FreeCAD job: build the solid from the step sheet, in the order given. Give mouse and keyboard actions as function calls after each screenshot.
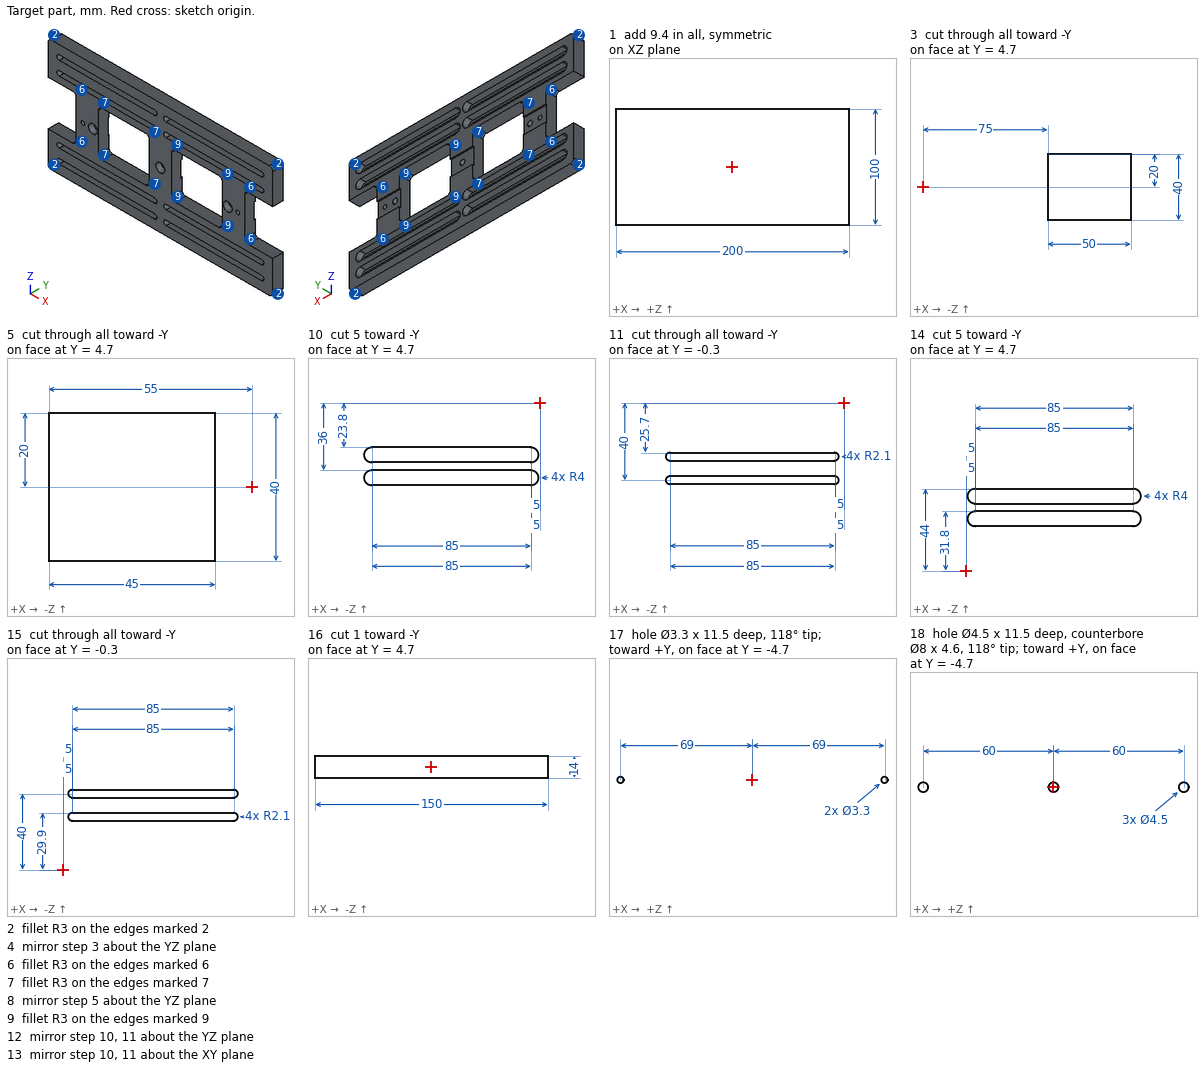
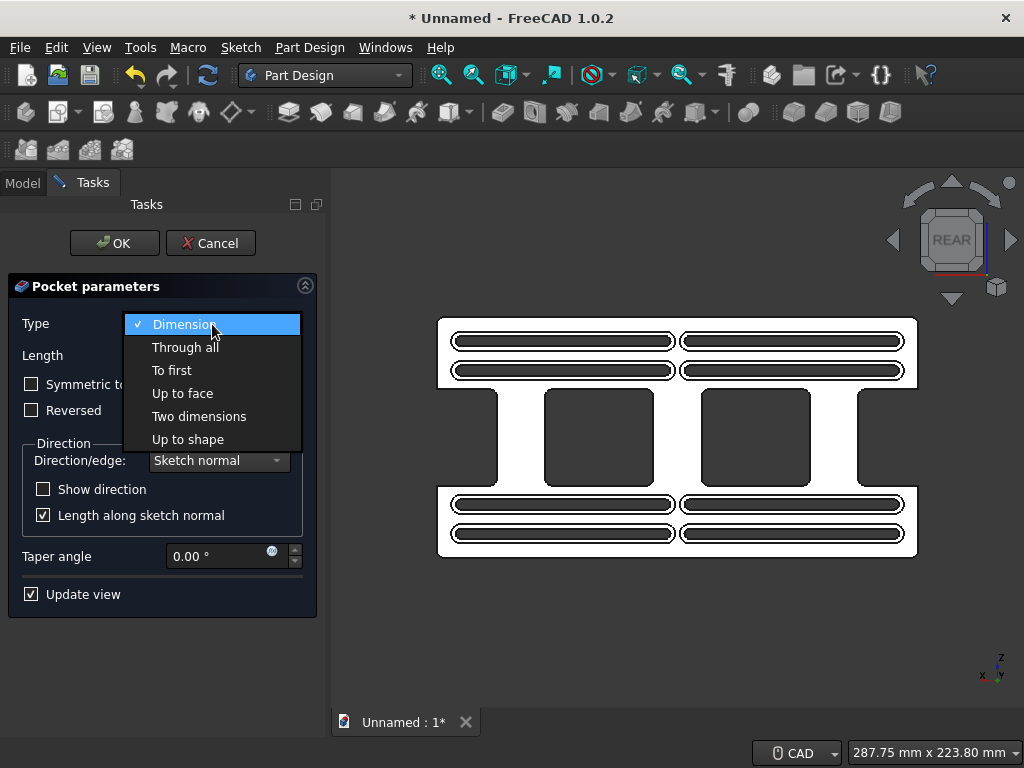
click(212, 348)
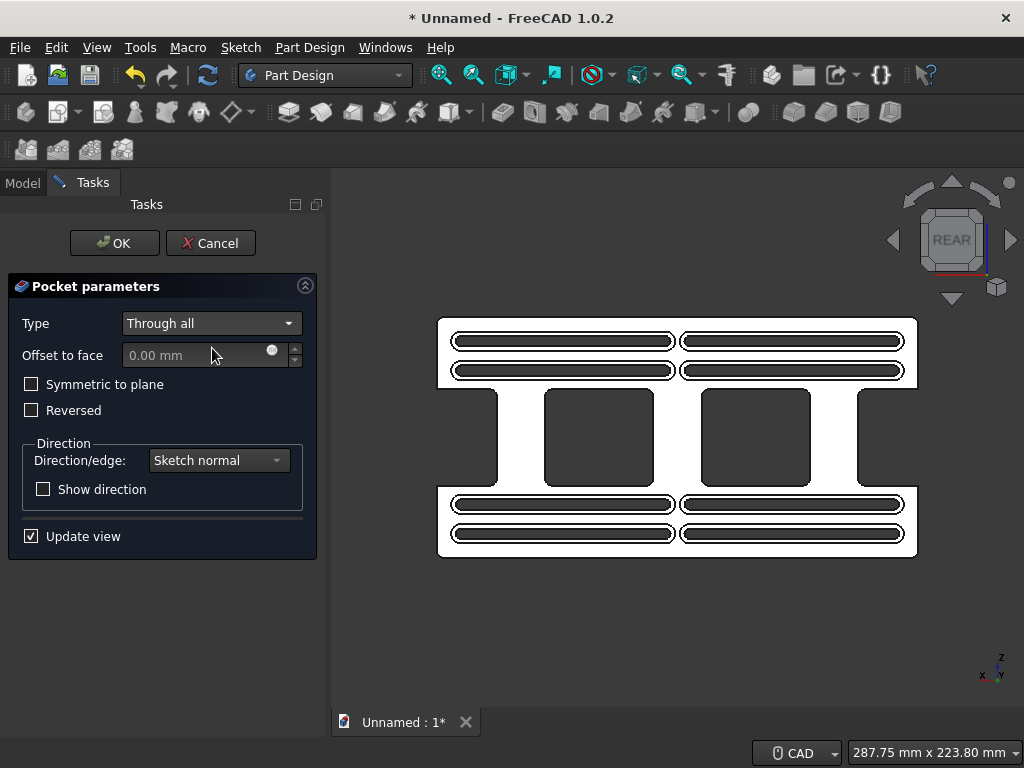
click(115, 243)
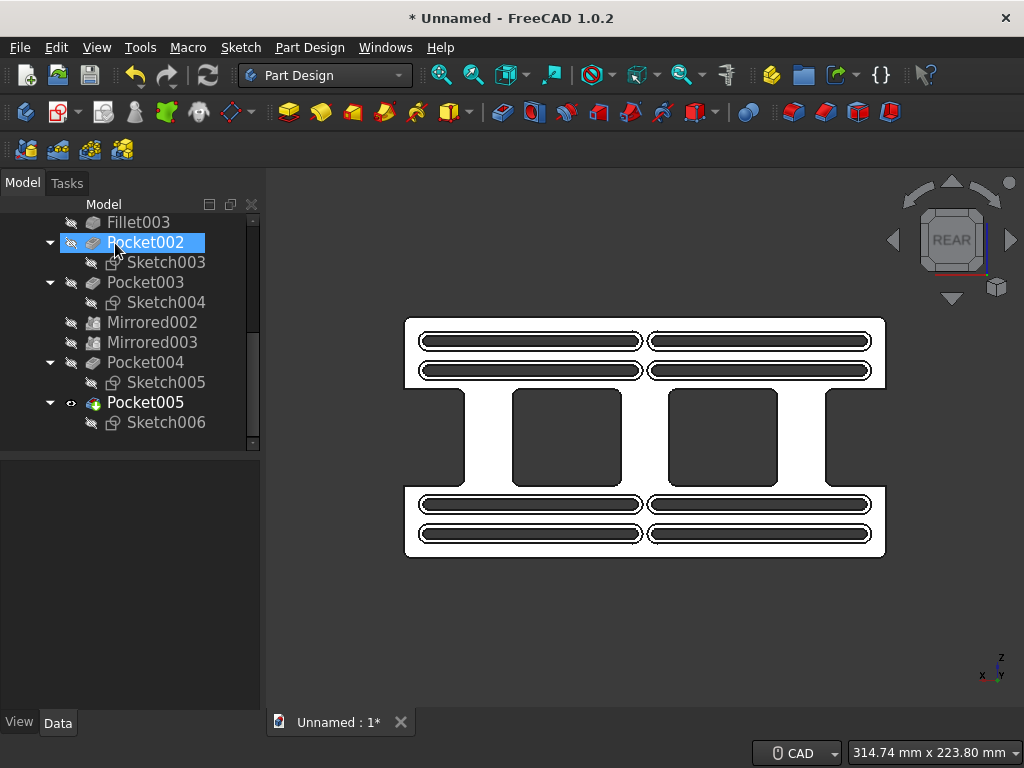
click(645, 437)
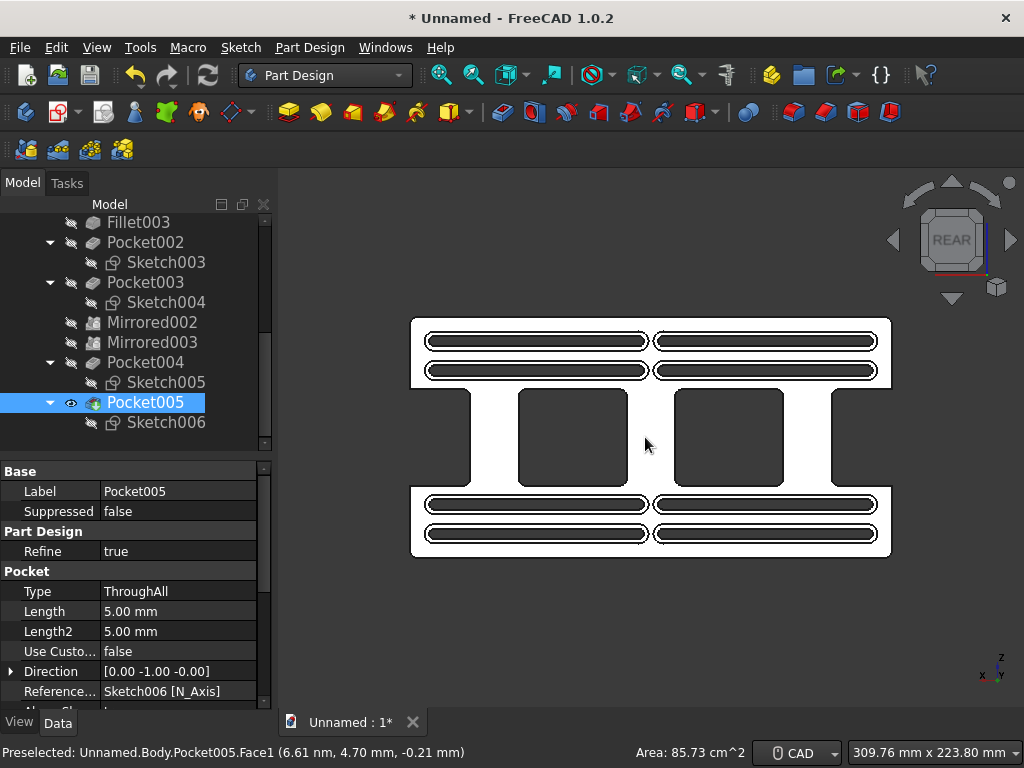
click(58, 112)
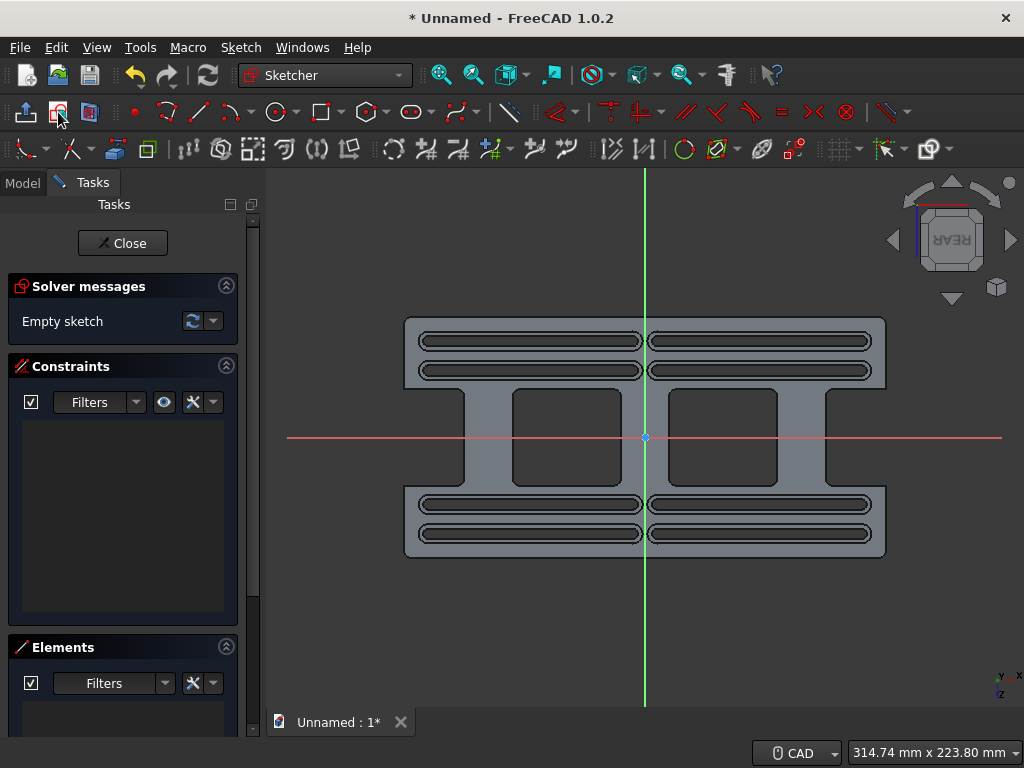
key(g)
key(v)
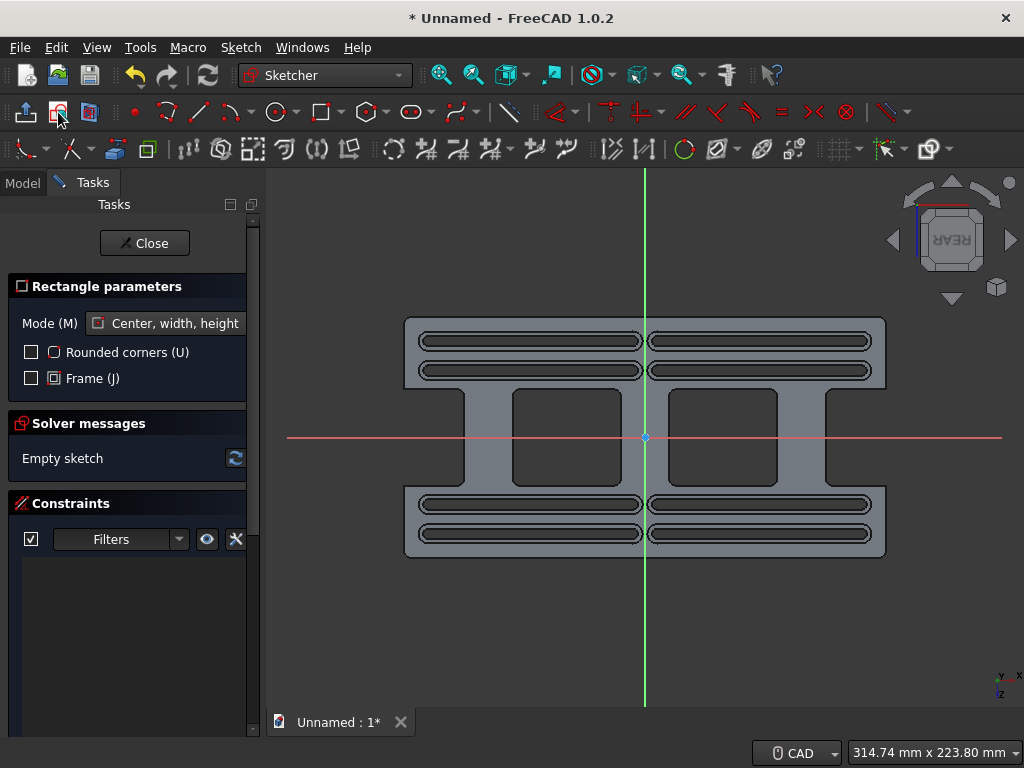
click(645, 437)
move(826, 421)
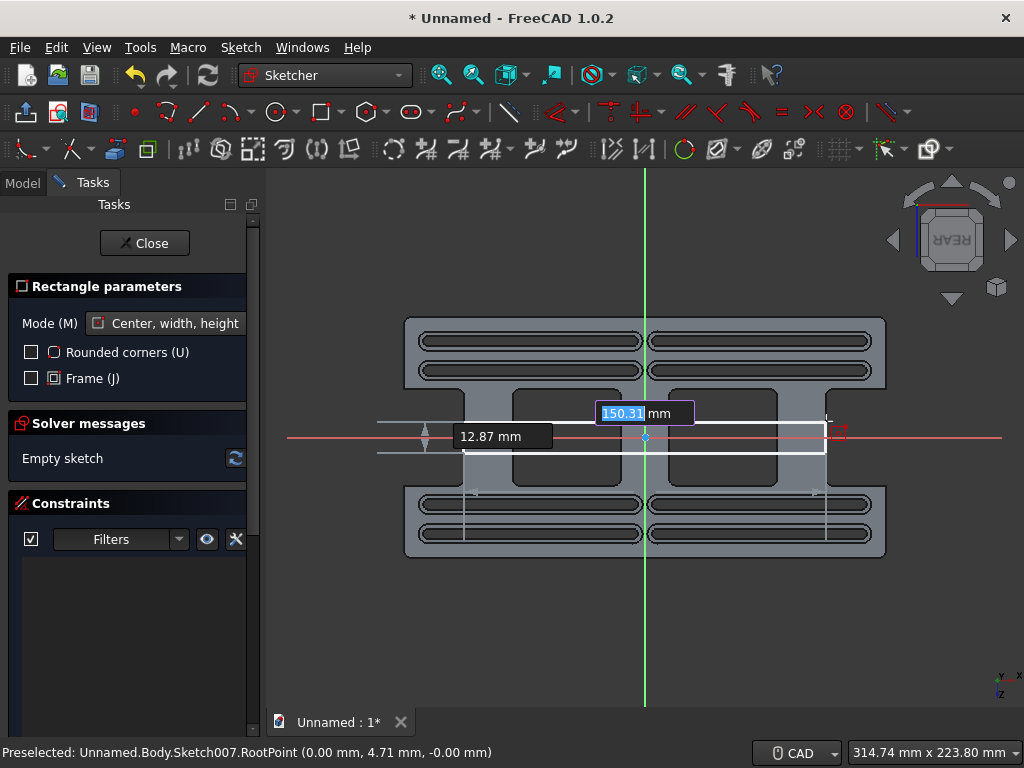
text(150)
key(Tab)
text(14)
key(Return)
key(Escape)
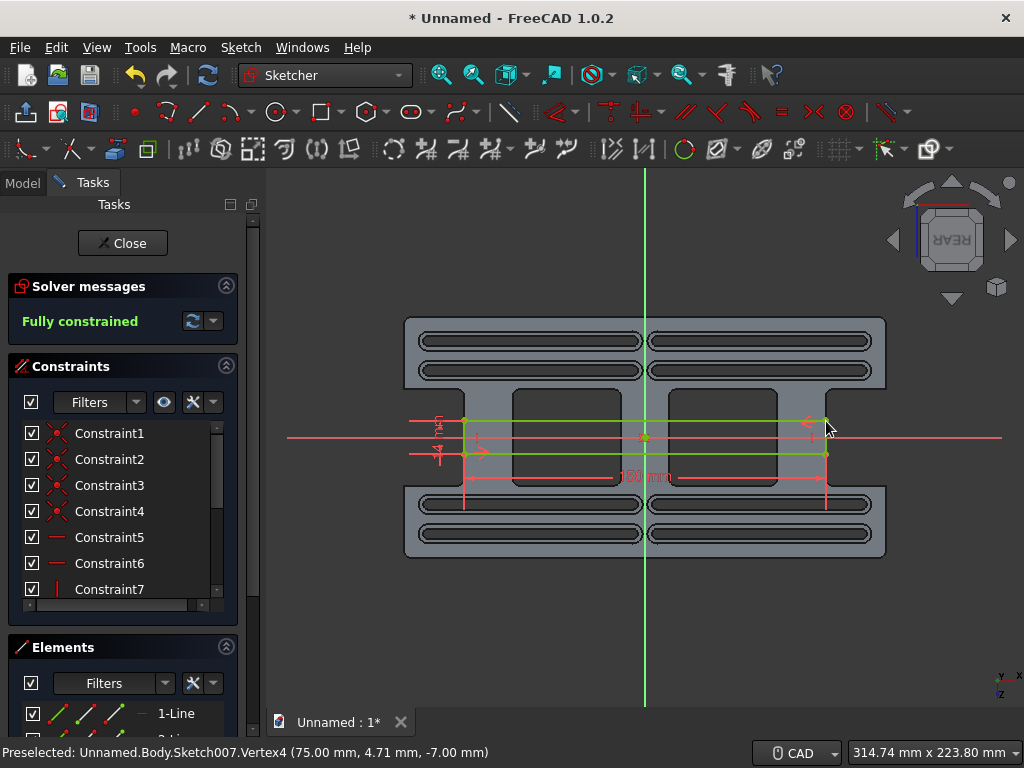
click(123, 243)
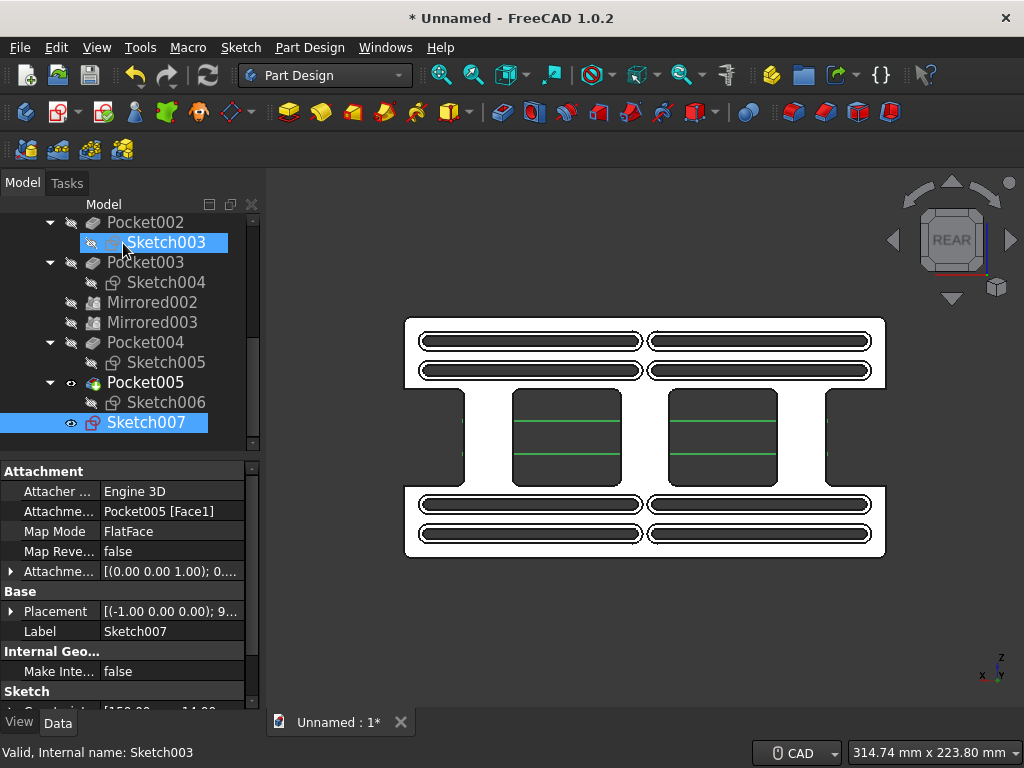
click(504, 112)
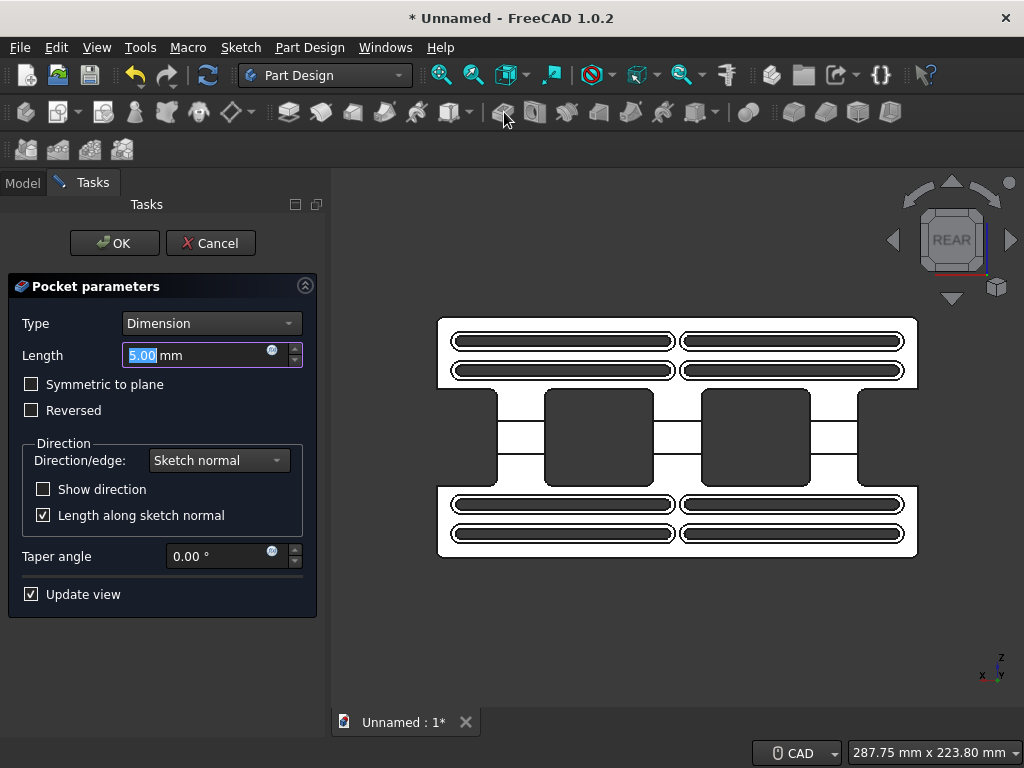
text(1)
key(Tab)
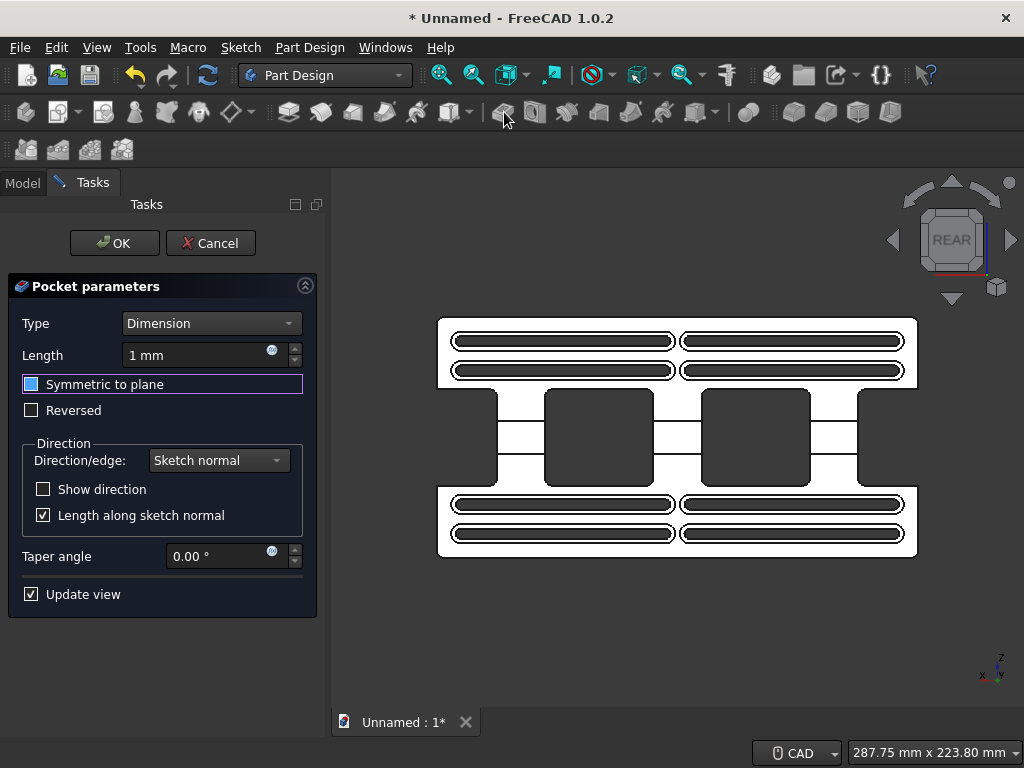
click(115, 243)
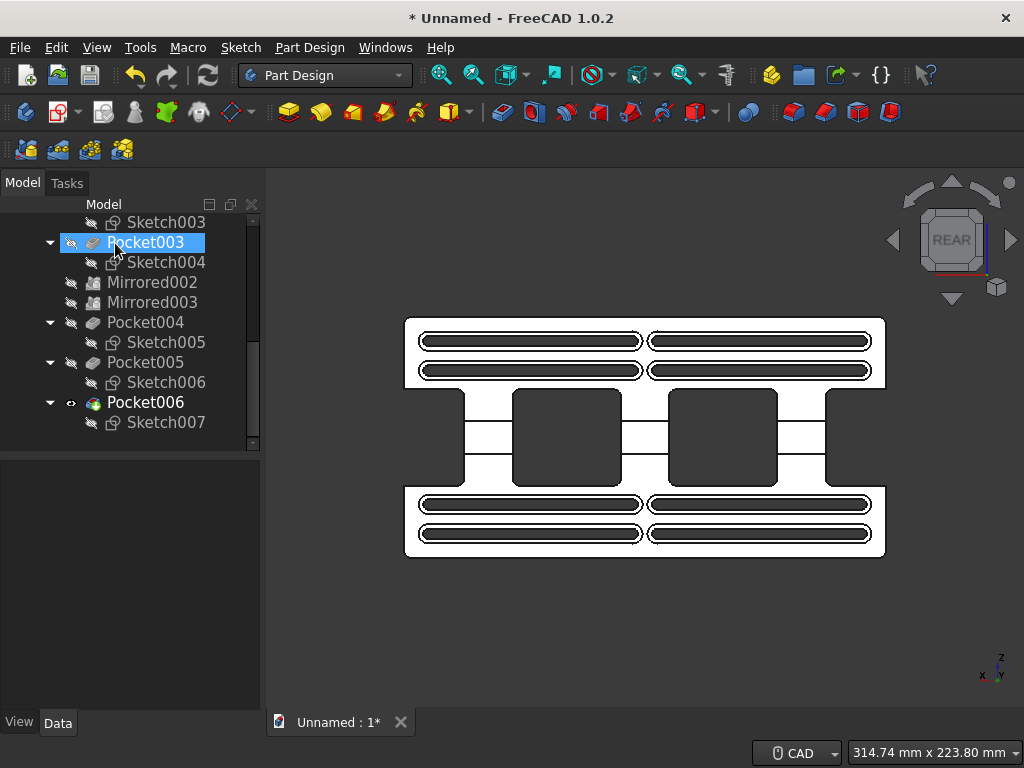
key(0)